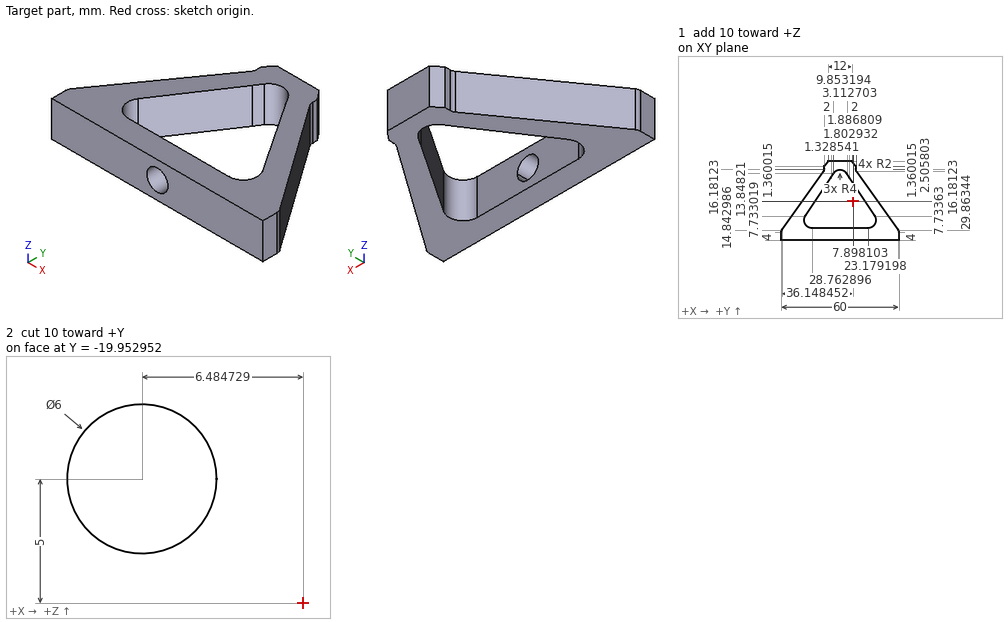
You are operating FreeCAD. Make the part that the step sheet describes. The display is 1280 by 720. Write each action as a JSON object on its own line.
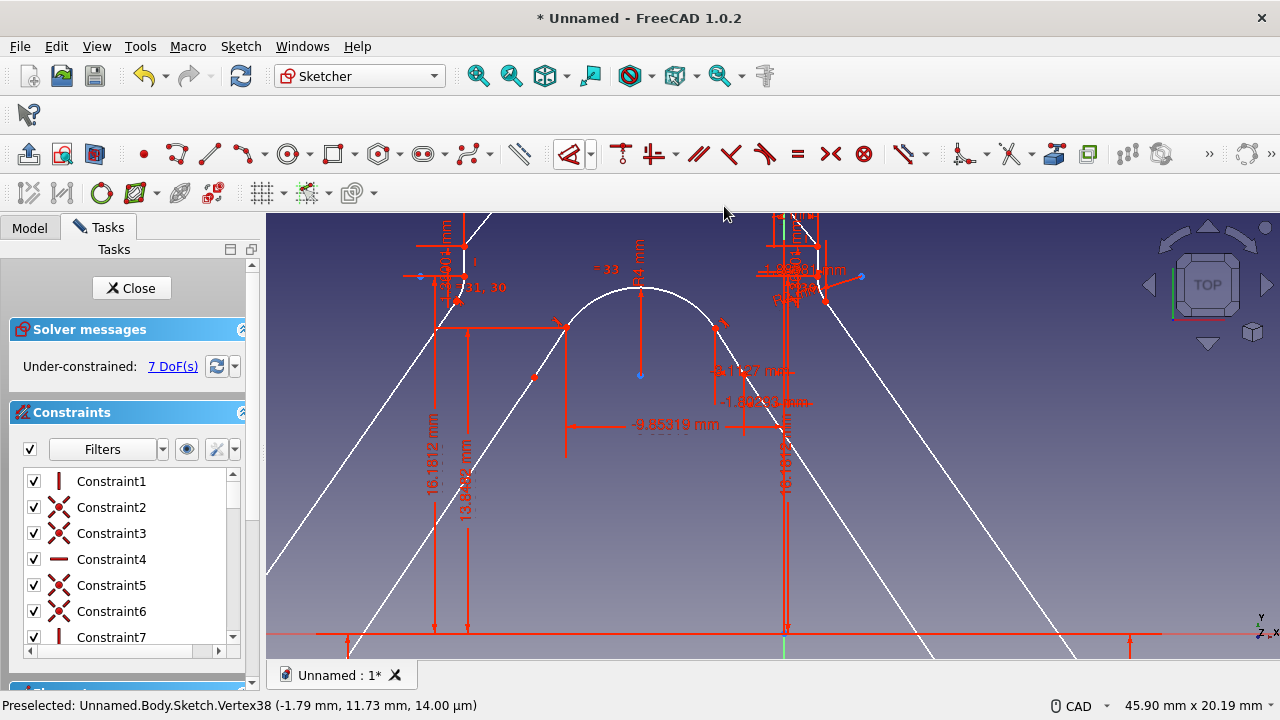
{"action": "scroll", "coordinate": [732, 351], "scroll_direction": "down", "scroll_amount": 6}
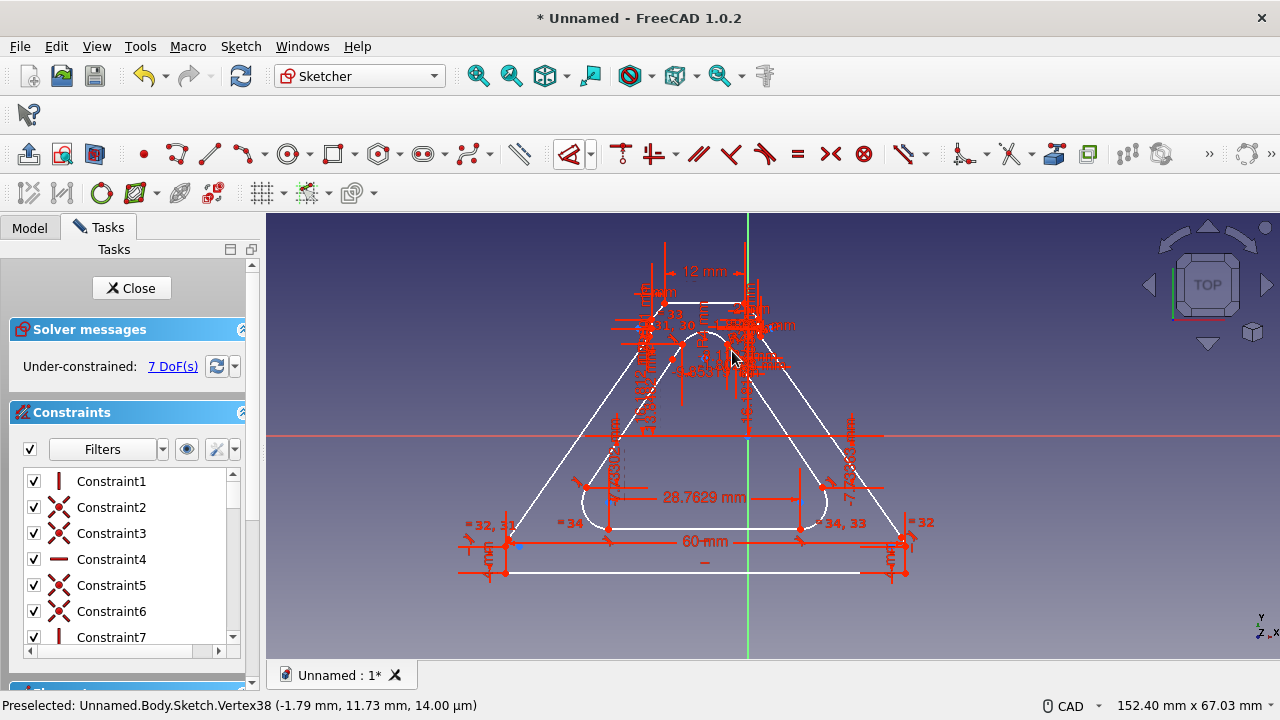
{"action": "left_click", "coordinate": [800, 529]}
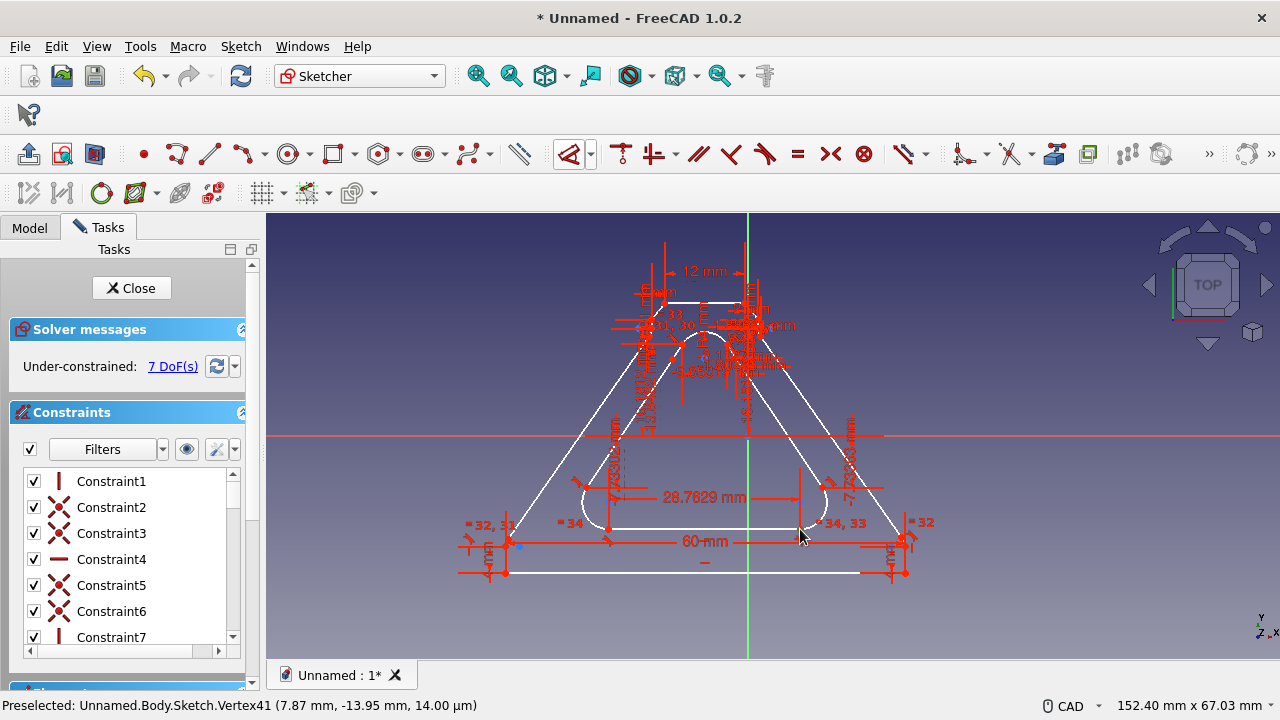
{"action": "left_click", "coordinate": [590, 154]}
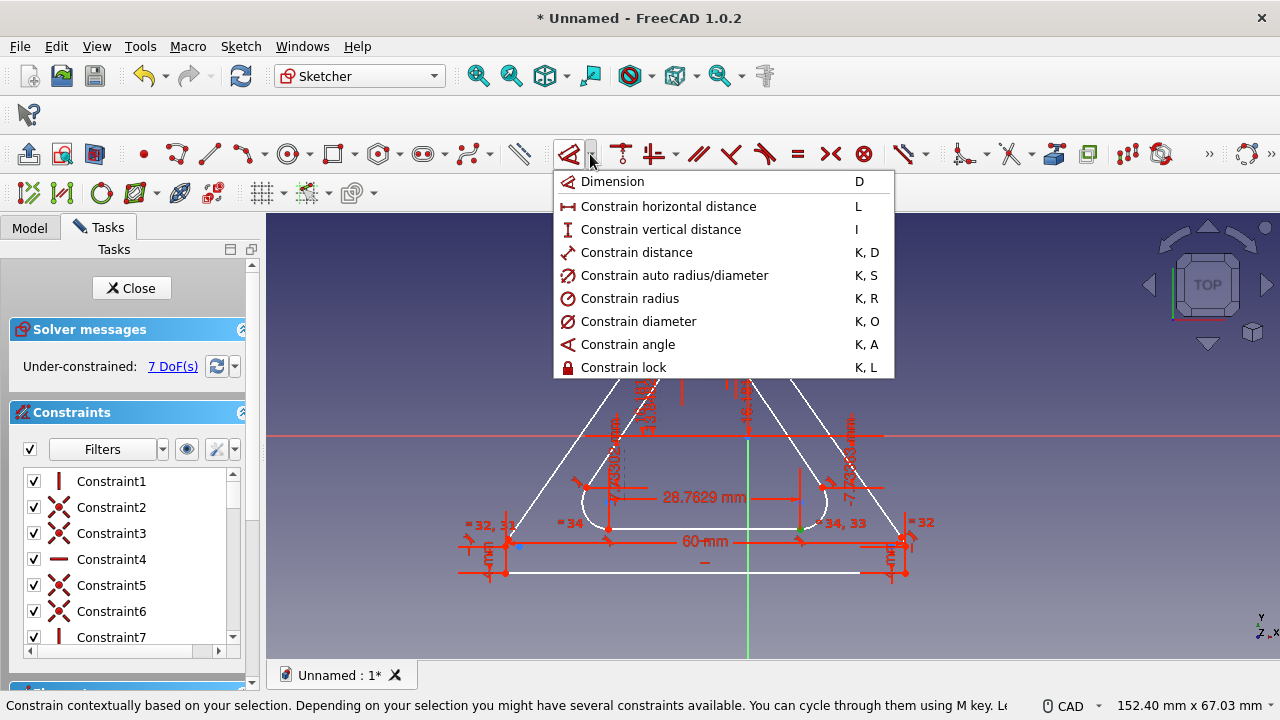
{"action": "left_click", "coordinate": [724, 206]}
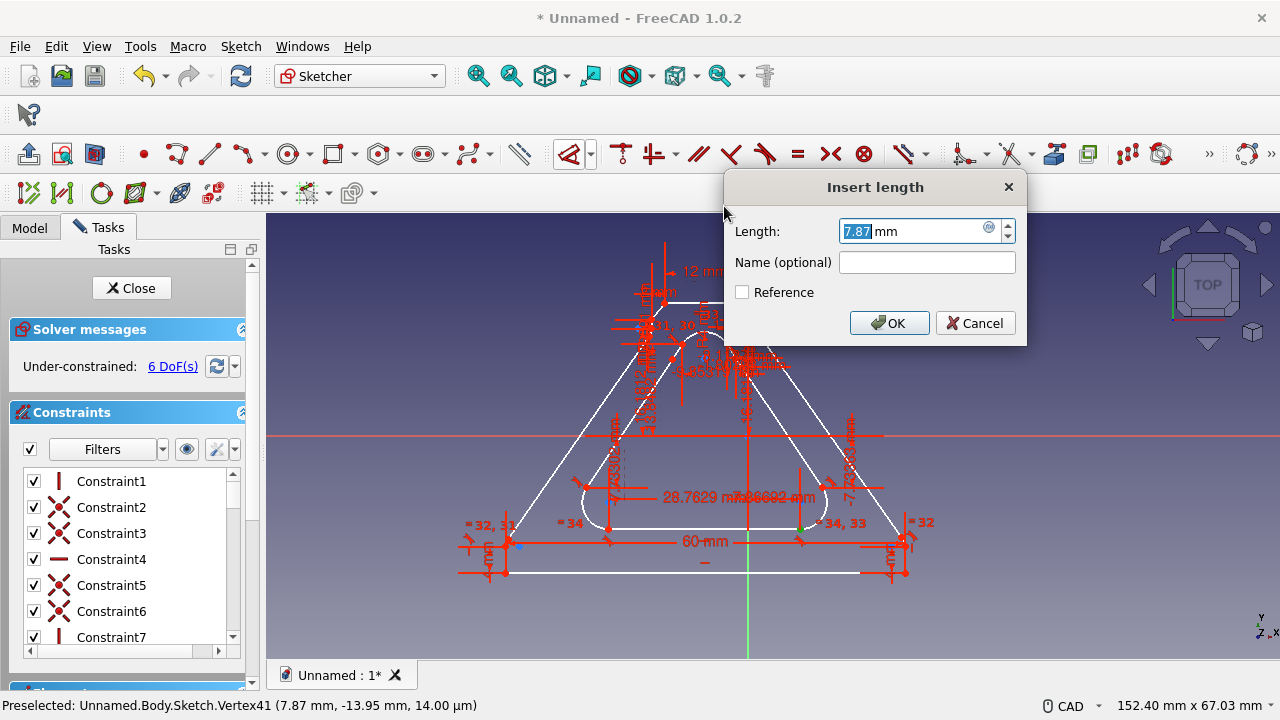
{"action": "type", "text": "7.898103"}
{"action": "key", "text": "Return"}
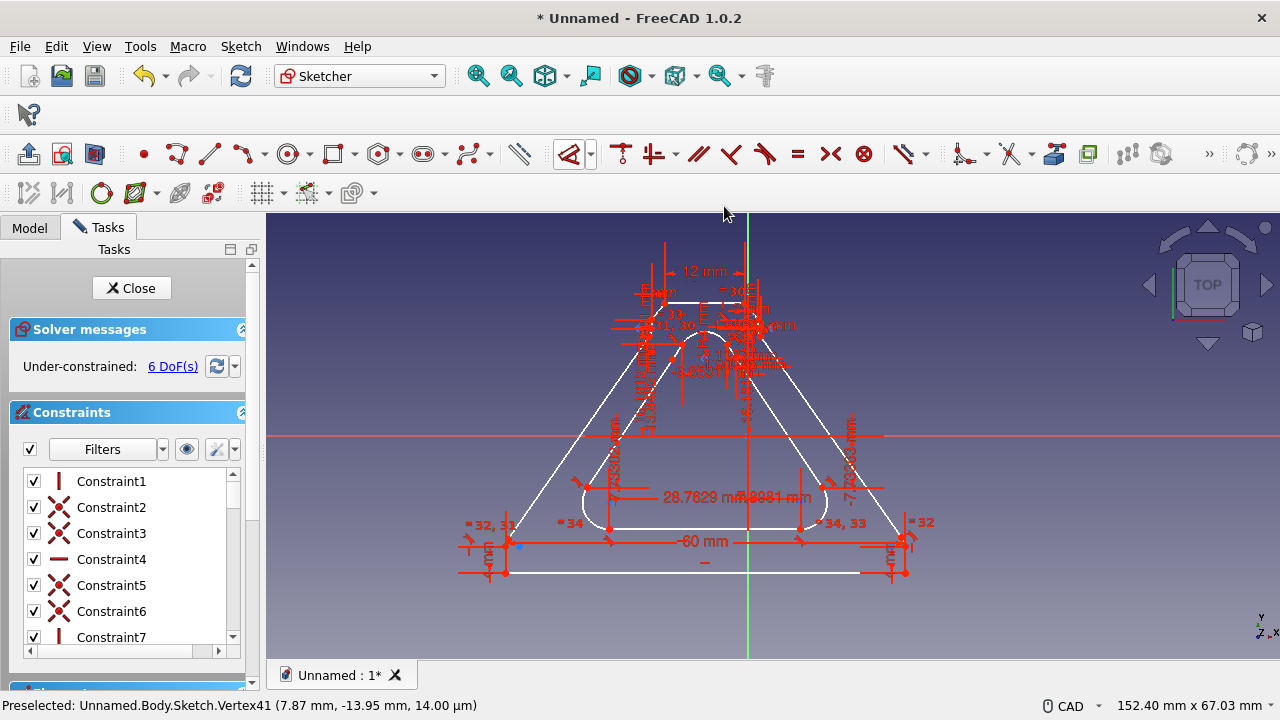
{"action": "left_click", "coordinate": [803, 397]}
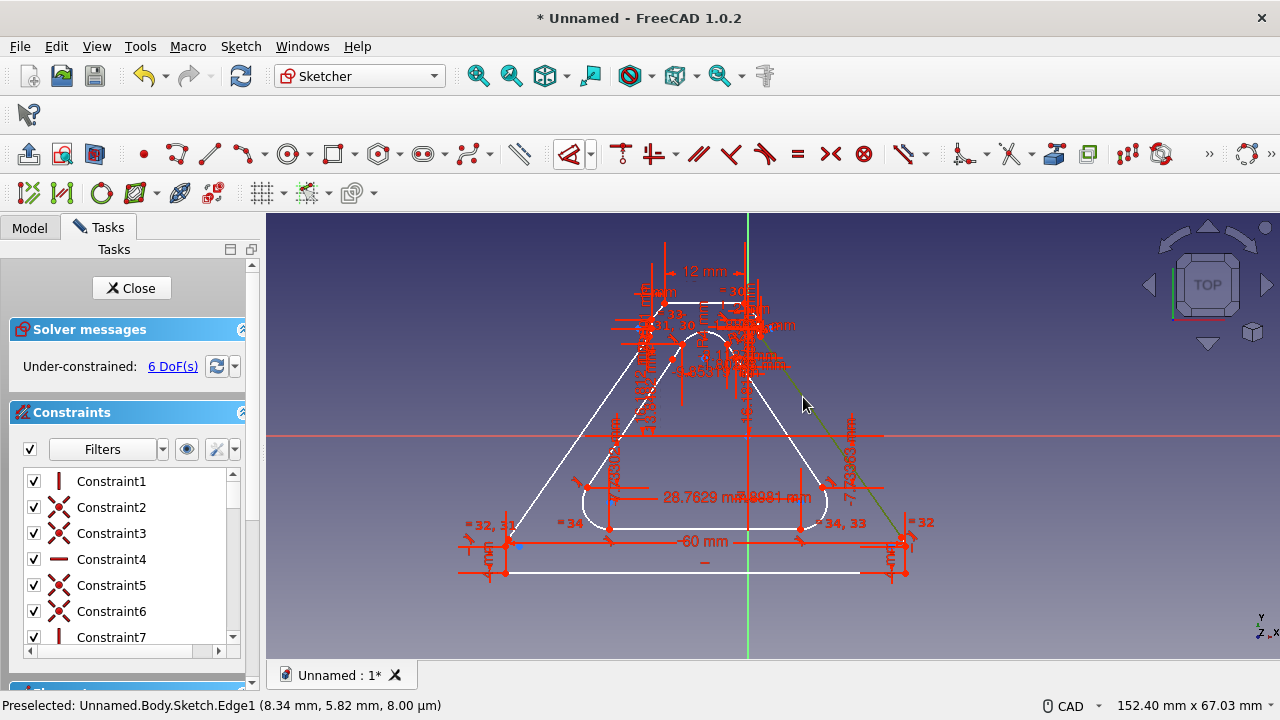
{"action": "left_click", "coordinate": [590, 154]}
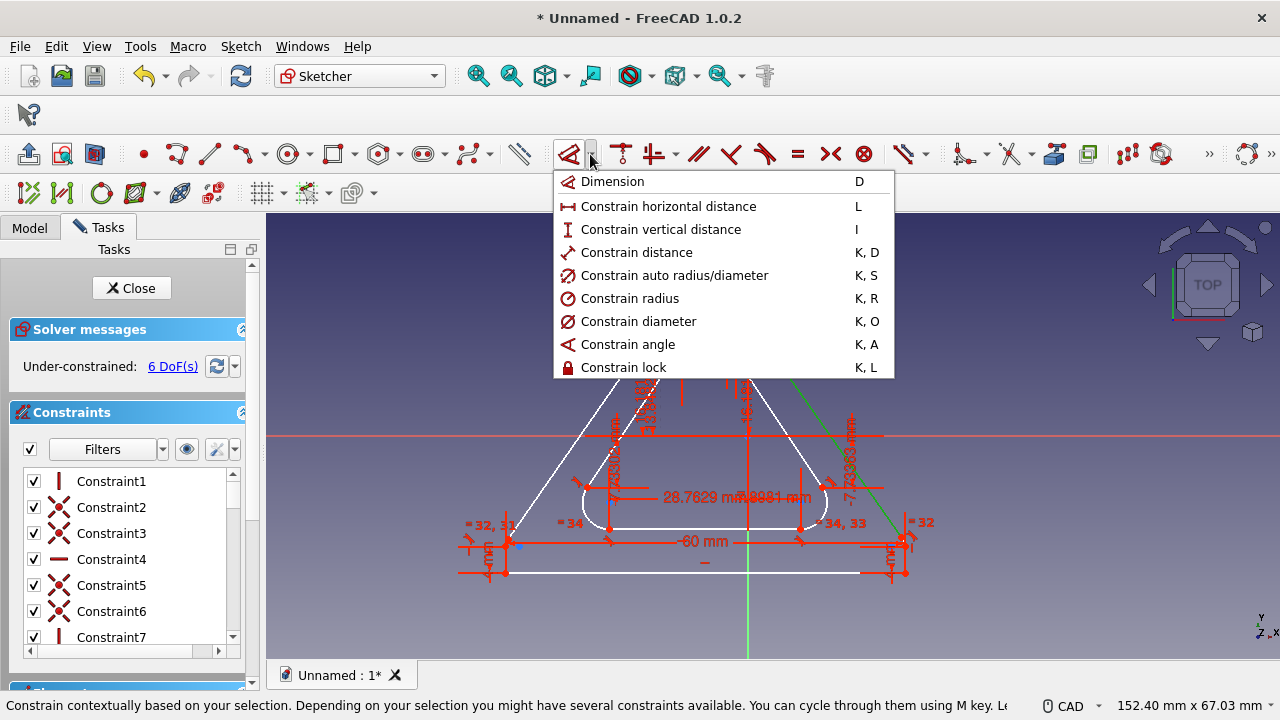
{"action": "left_click", "coordinate": [724, 230]}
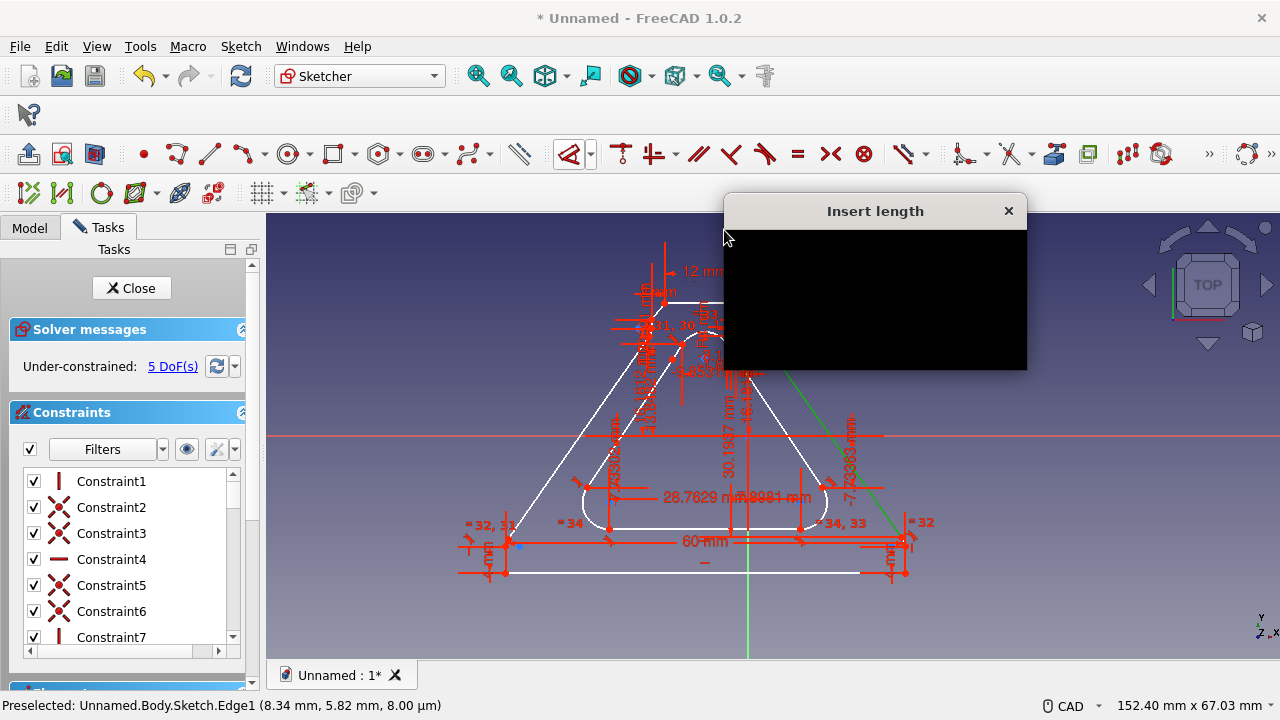
{"action": "type", "text": "29.86344"}
{"action": "key", "text": "Return"}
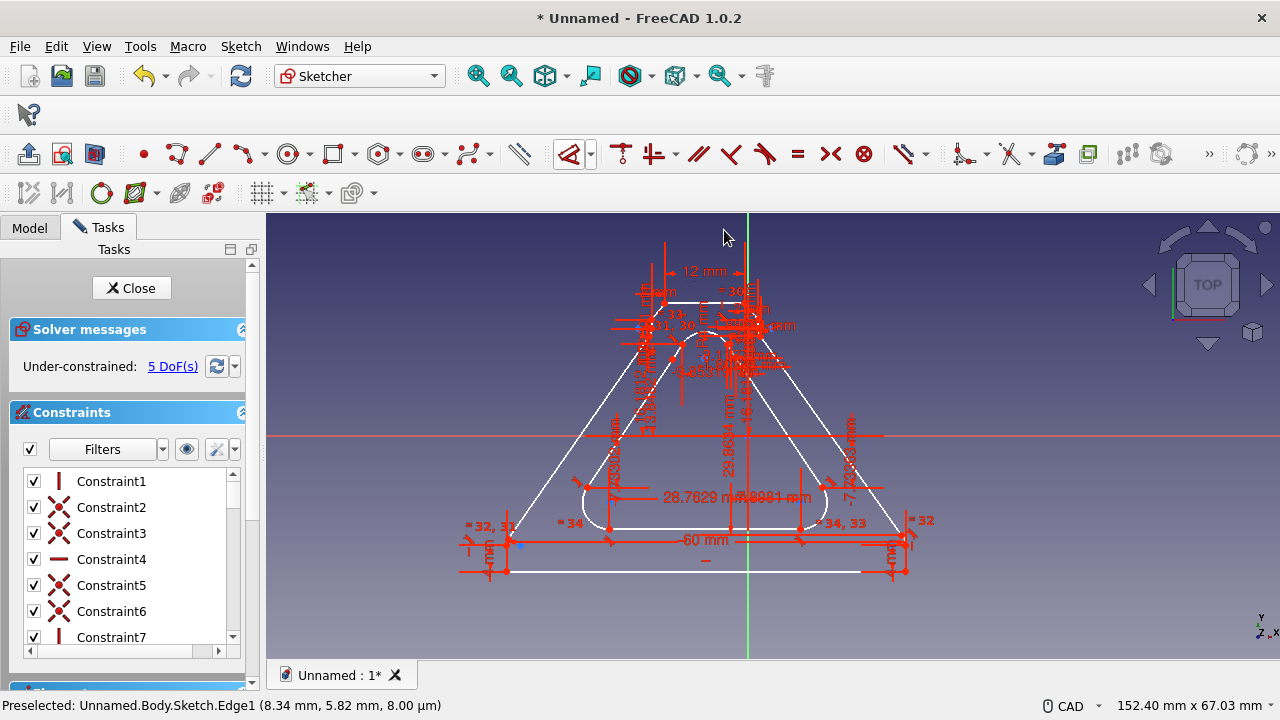
{"action": "scroll", "coordinate": [751, 311], "scroll_direction": "up", "scroll_amount": 5}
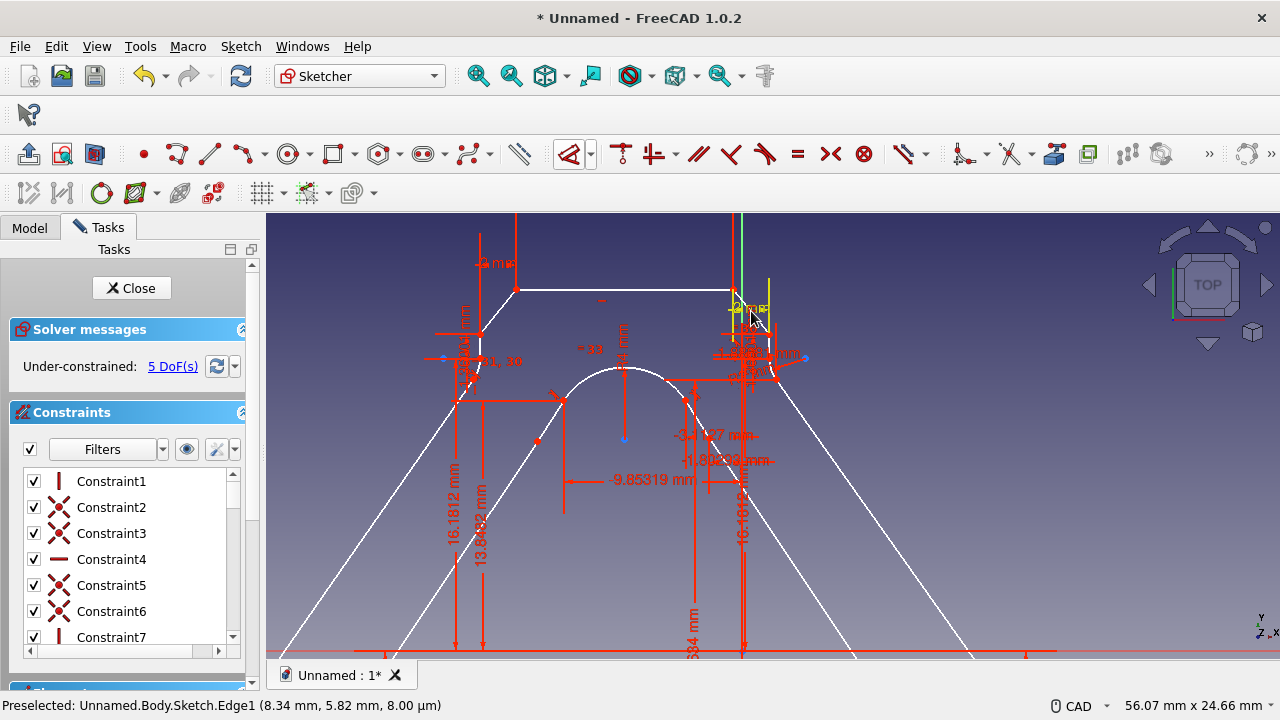
{"action": "left_click", "coordinate": [762, 325]}